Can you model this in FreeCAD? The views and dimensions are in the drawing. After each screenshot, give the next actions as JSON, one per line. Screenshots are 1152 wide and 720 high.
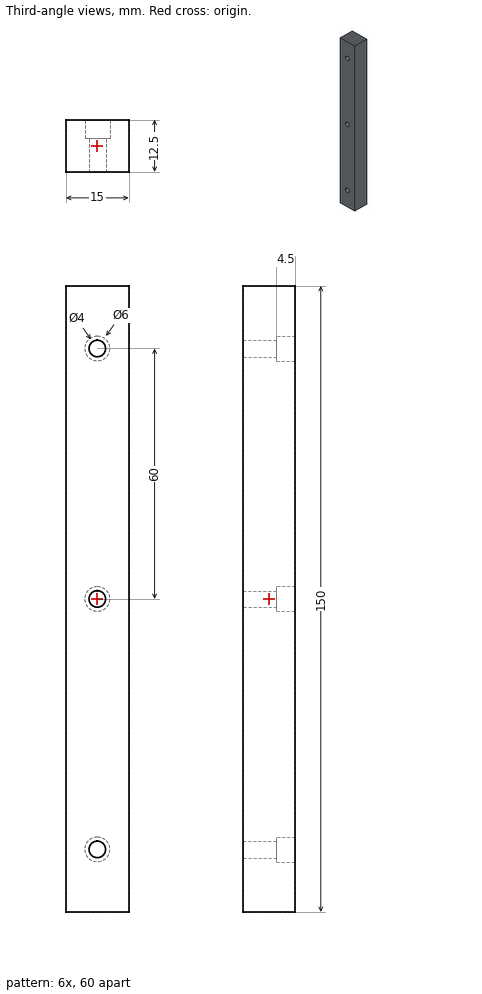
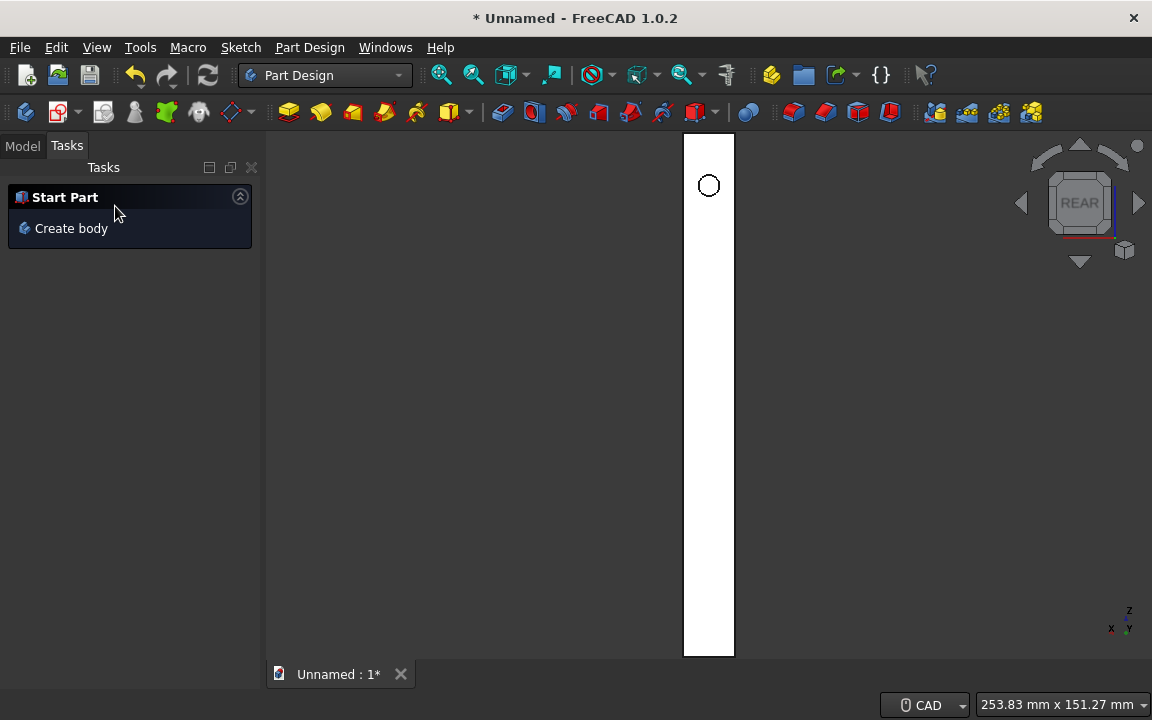
{"action": "left_click", "coordinate": [709, 244]}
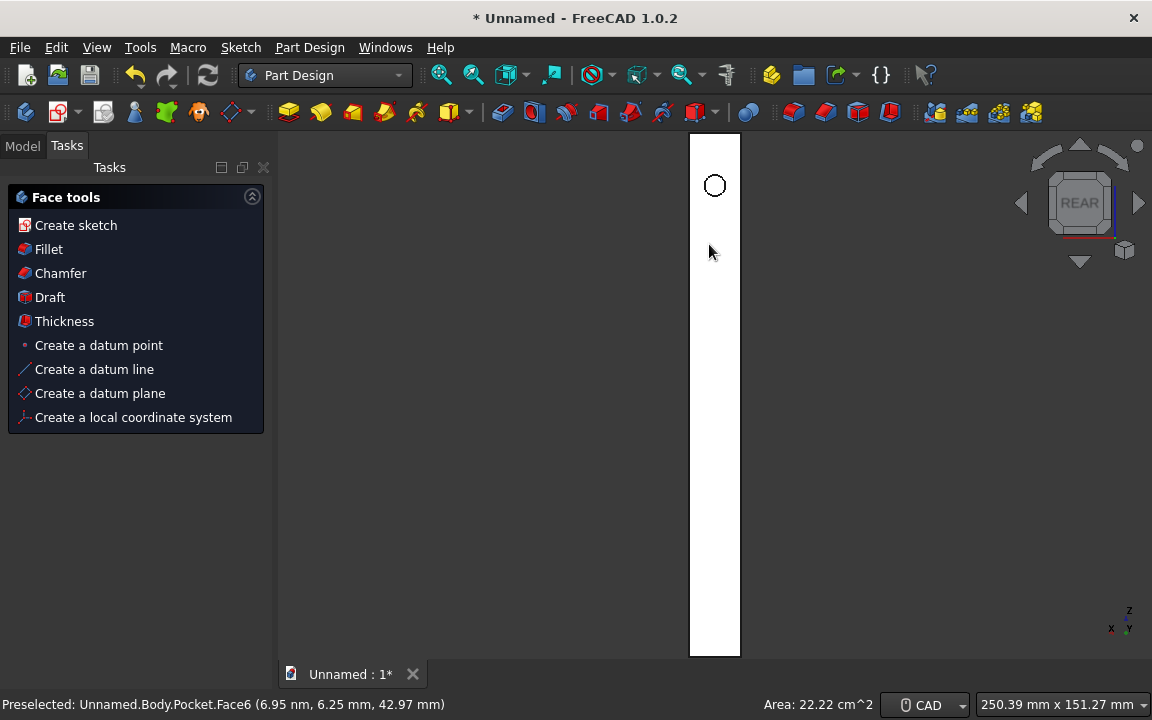
{"action": "left_click", "coordinate": [58, 112]}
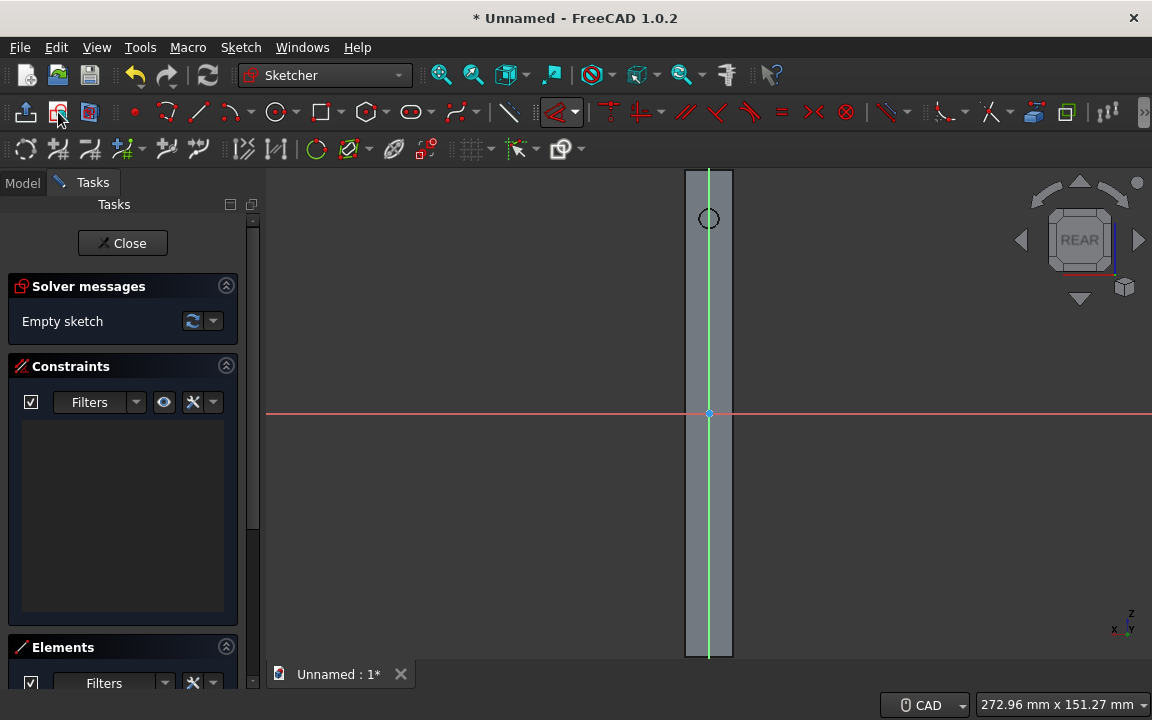
{"action": "scroll", "coordinate": [713, 209], "scroll_direction": "up", "scroll_amount": 15}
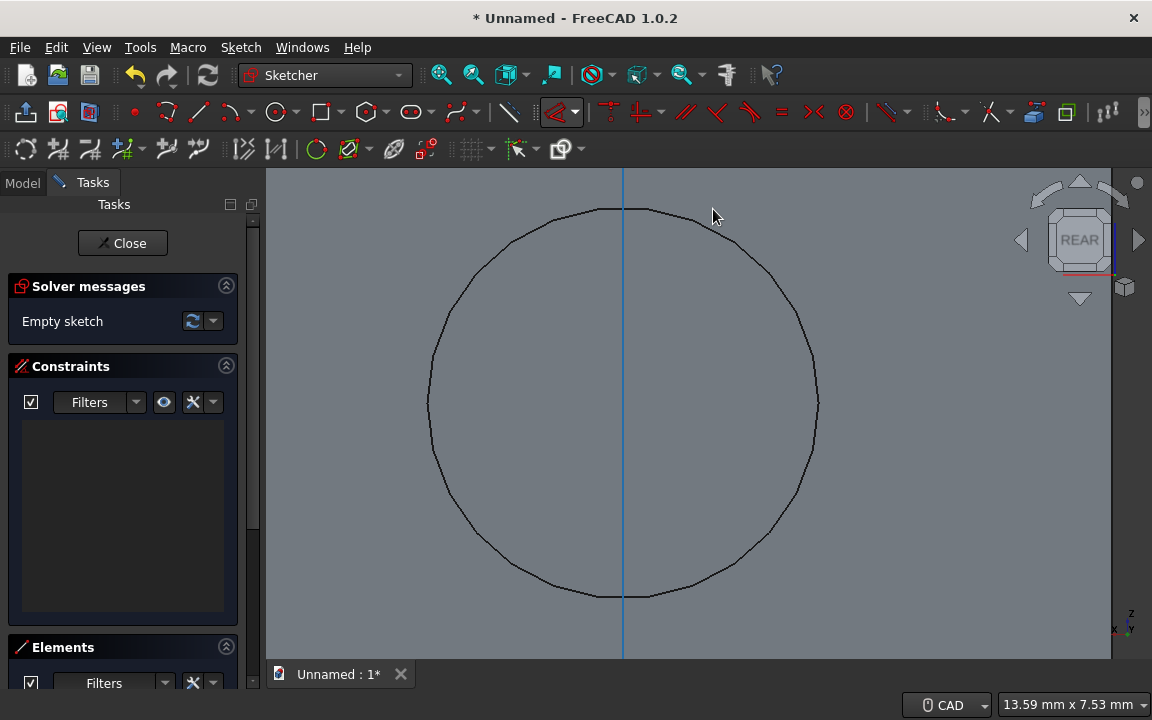
{"action": "key", "text": "g c"}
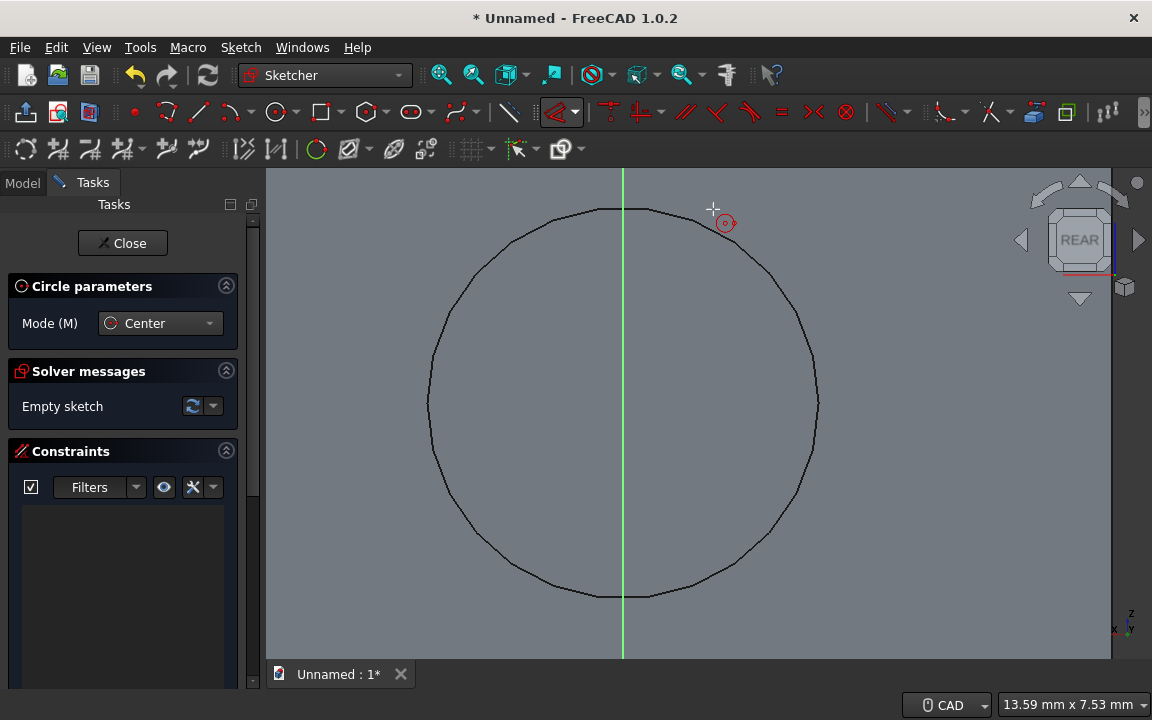
{"action": "left_click", "coordinate": [623, 403]}
{"action": "left_click", "coordinate": [715, 311]}
{"action": "key", "text": "Escape"}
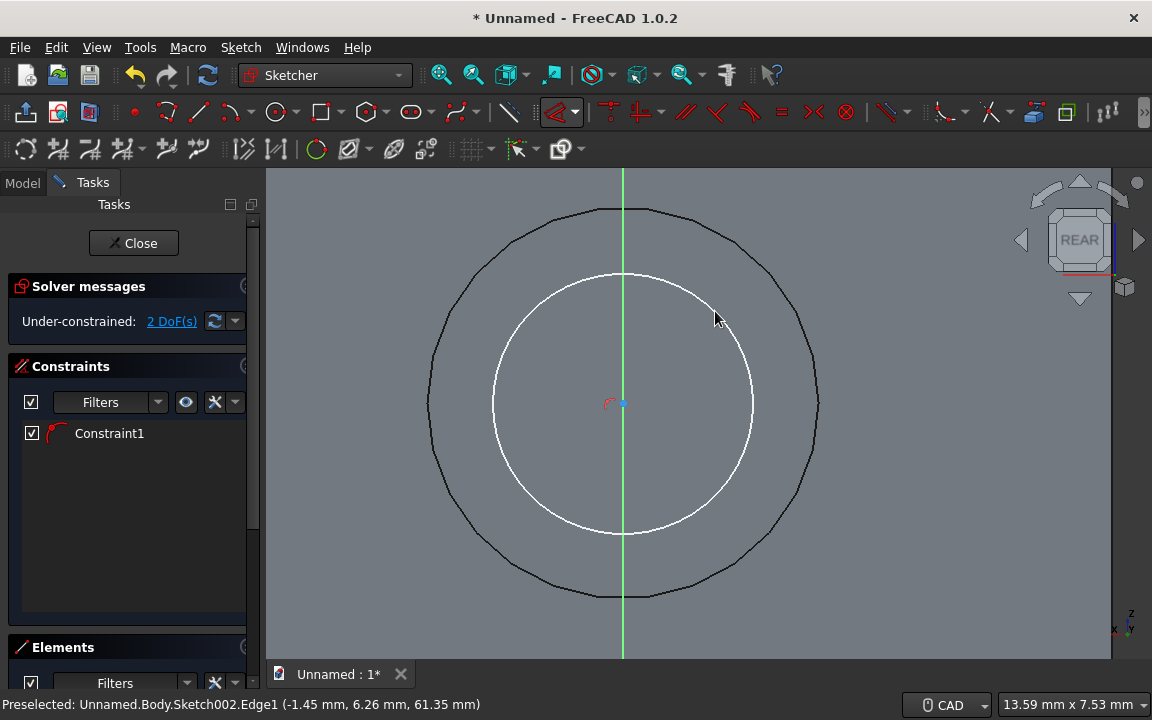
{"action": "left_click", "coordinate": [715, 312]}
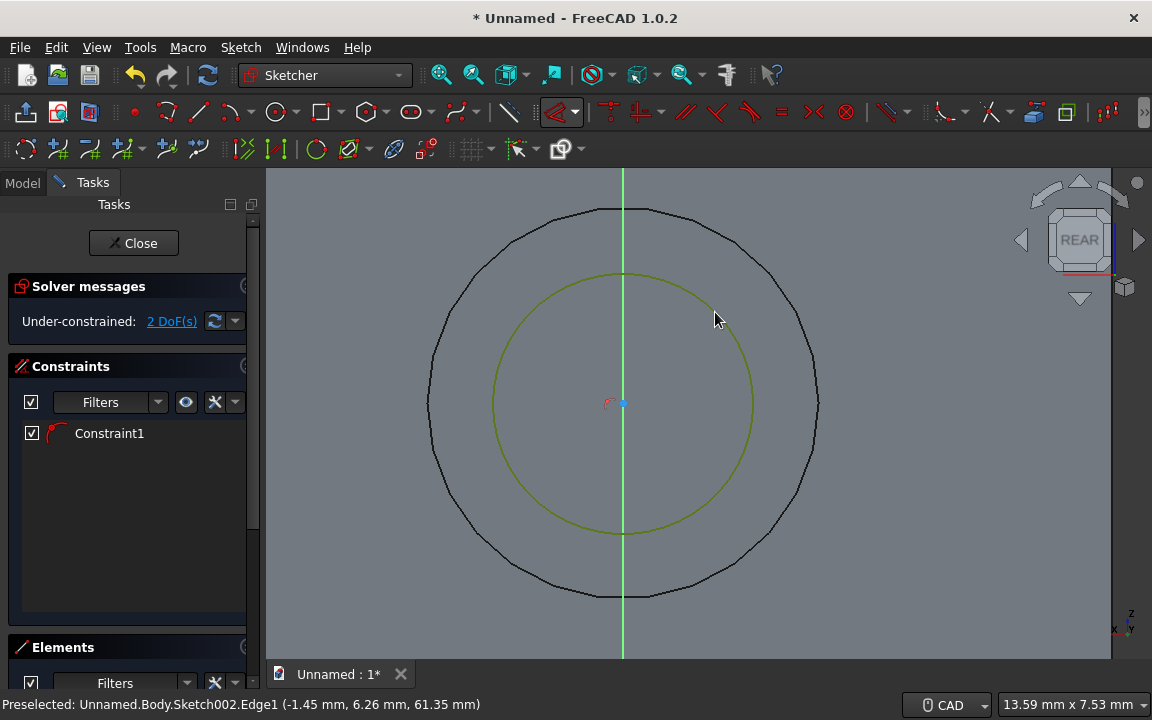
{"action": "key", "text": "k o"}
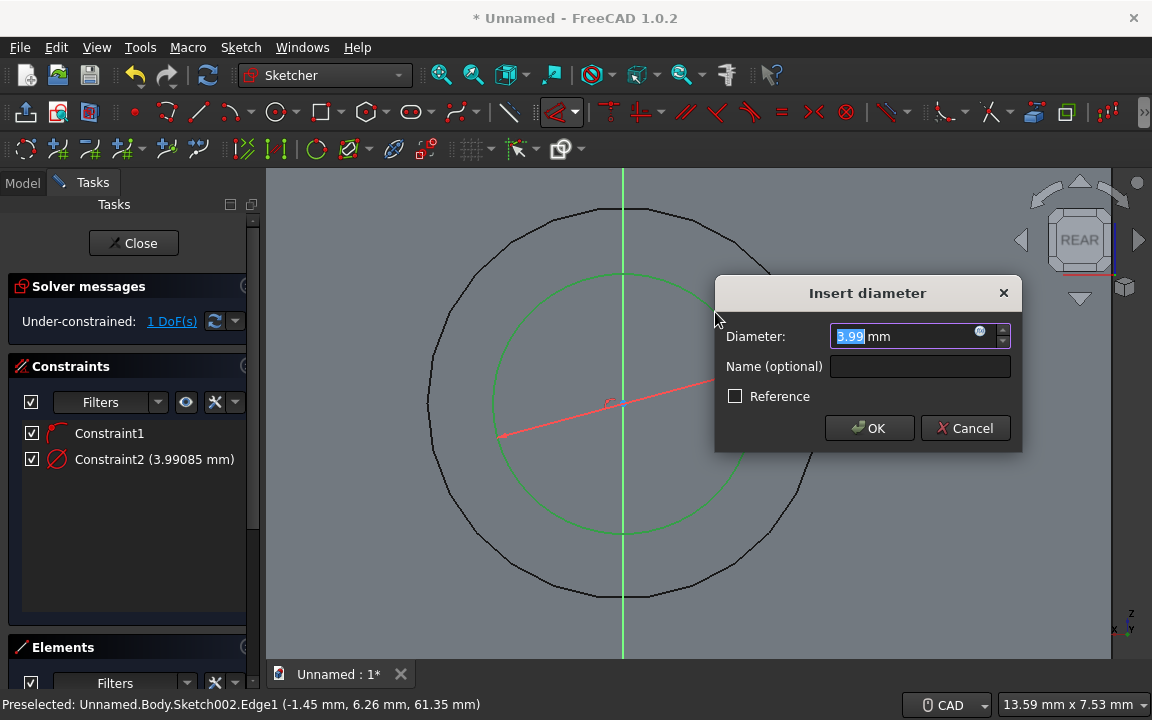
{"action": "type", "text": "4"}
{"action": "key", "text": "Return"}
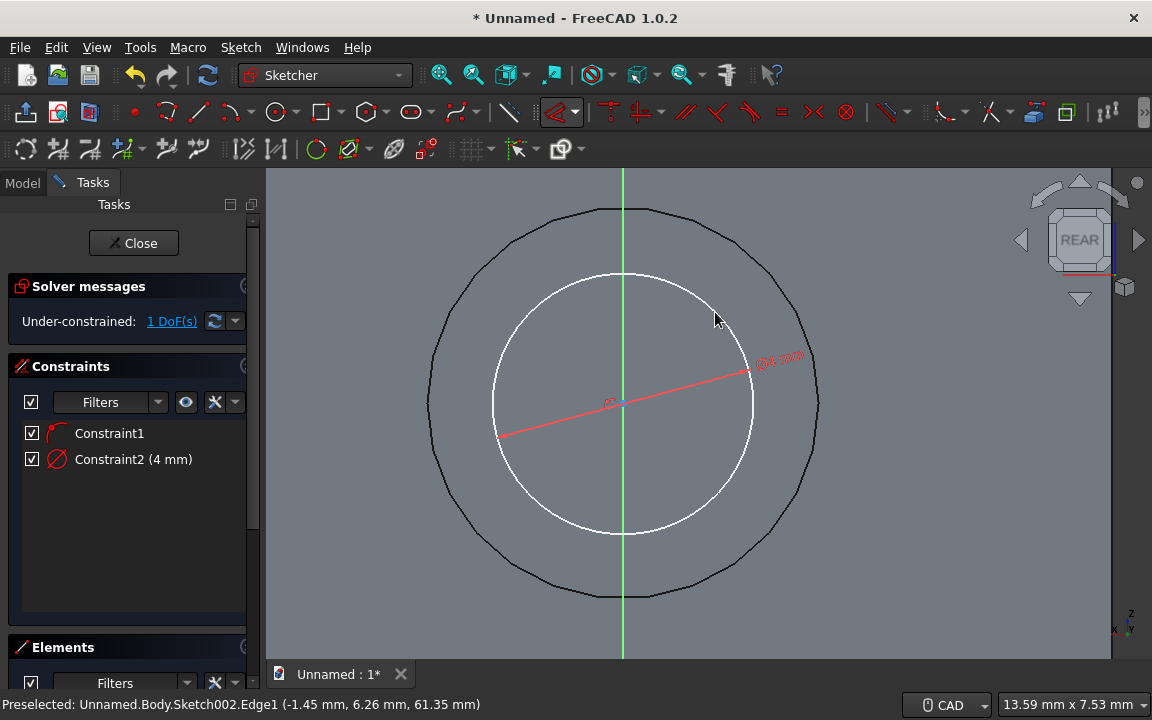
{"action": "left_click", "coordinate": [623, 404]}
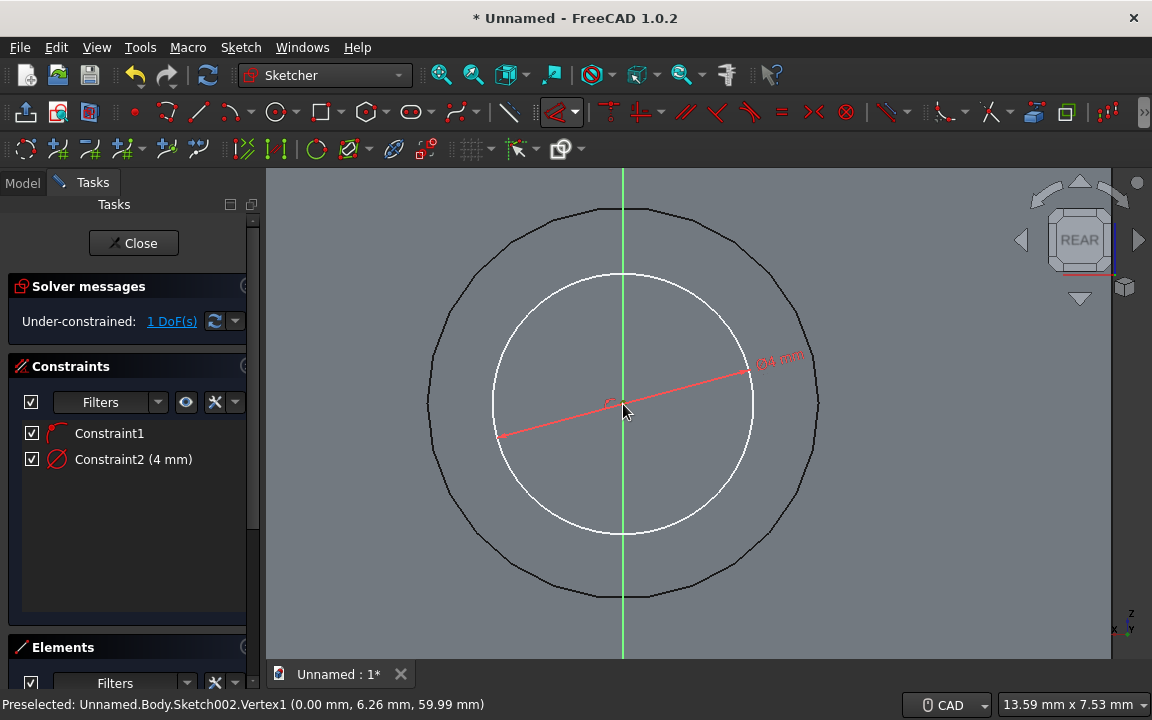
{"action": "left_click", "coordinate": [578, 112]}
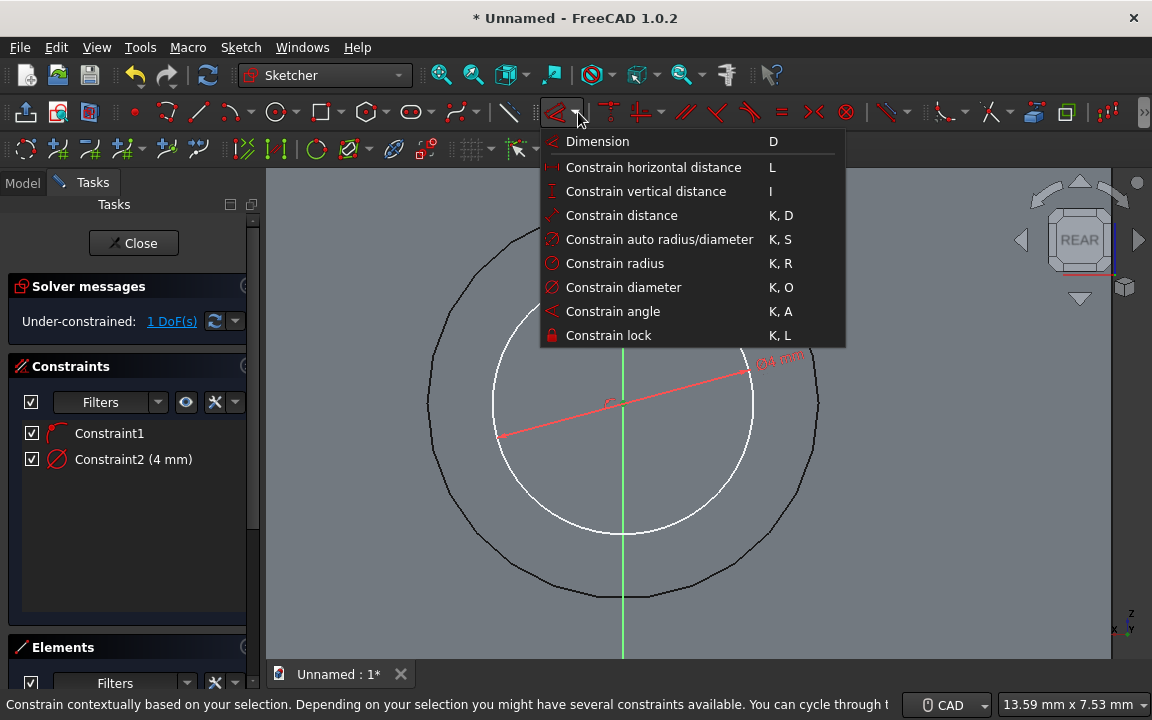
{"action": "left_click", "coordinate": [693, 191]}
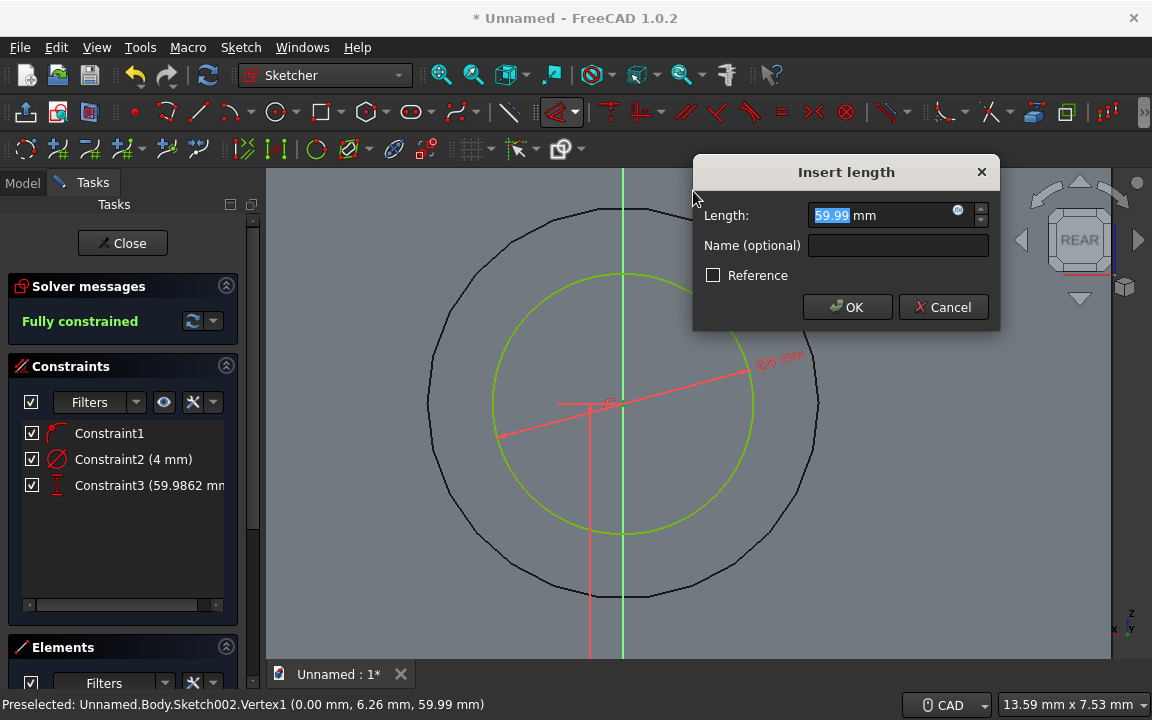
{"action": "type", "text": "60"}
{"action": "key", "text": "Return"}